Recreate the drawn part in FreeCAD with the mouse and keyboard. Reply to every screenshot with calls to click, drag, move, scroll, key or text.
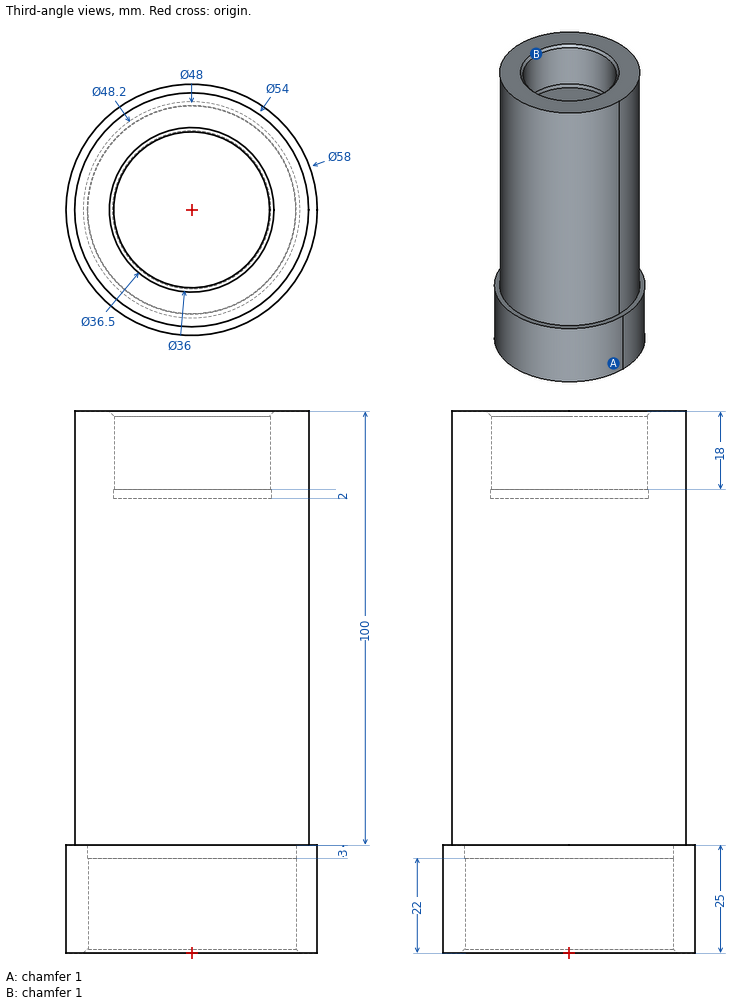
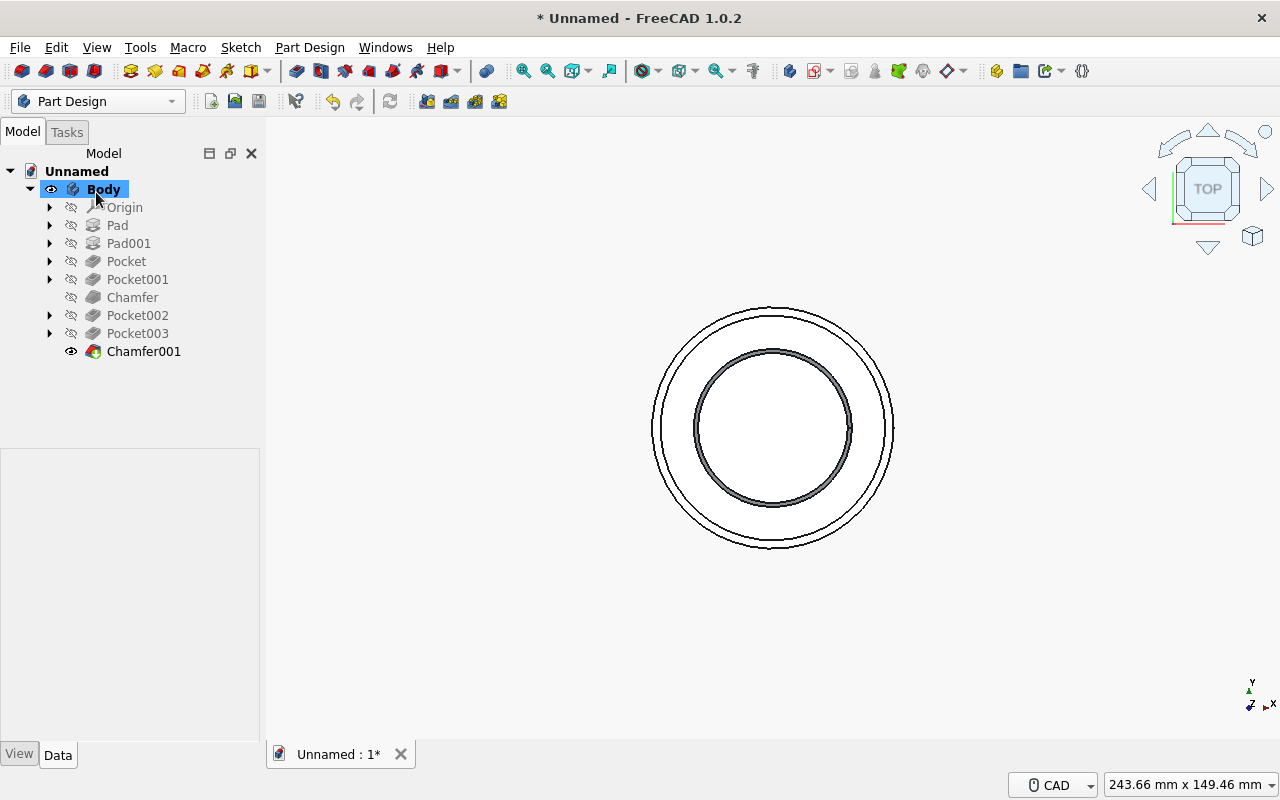
key(0)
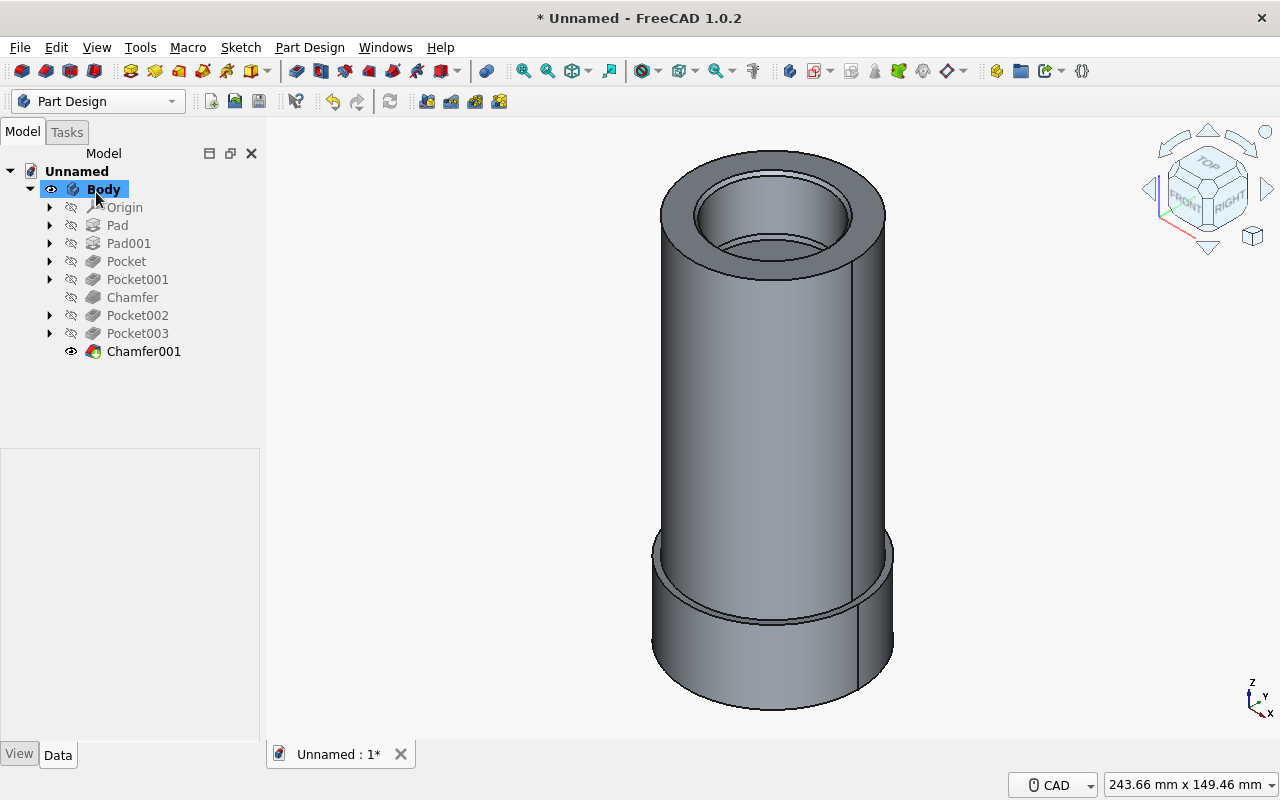
click(524, 72)